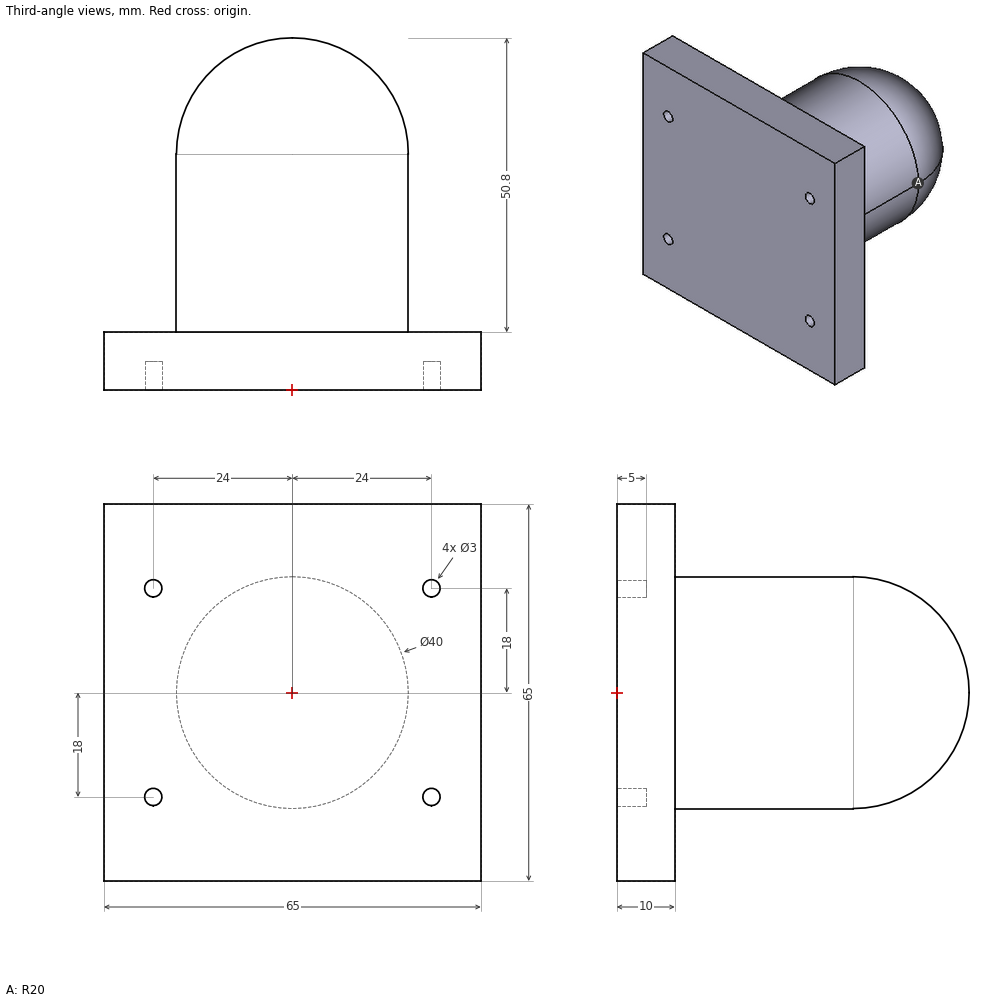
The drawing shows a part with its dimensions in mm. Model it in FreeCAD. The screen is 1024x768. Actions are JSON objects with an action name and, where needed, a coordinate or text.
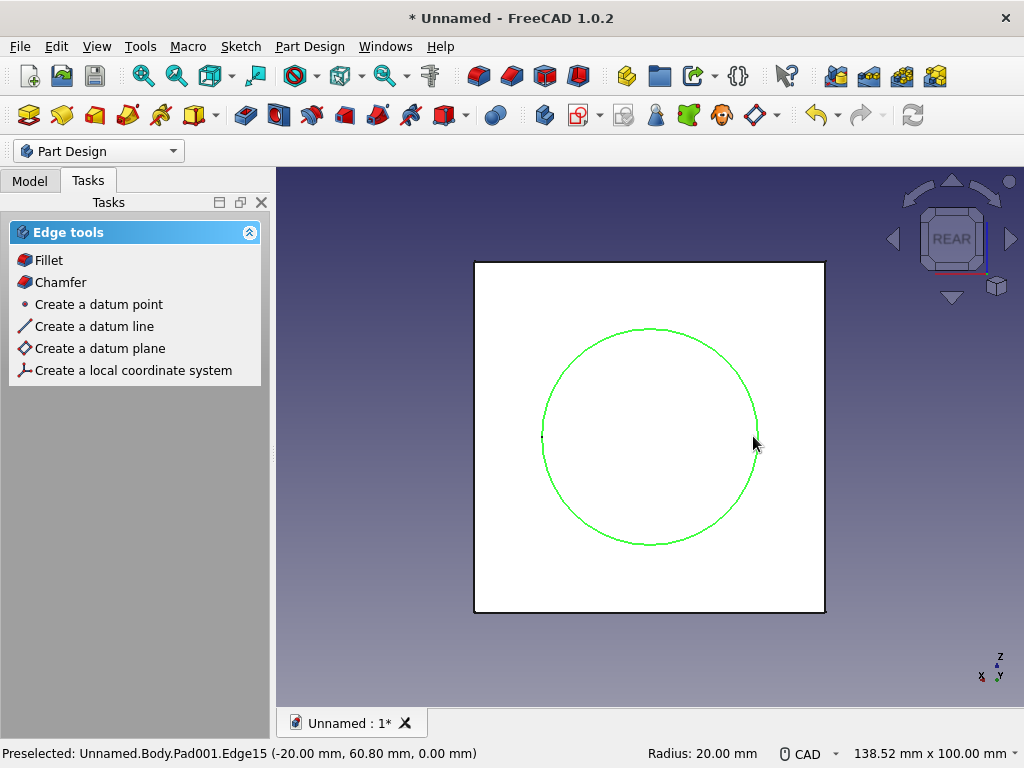
{"action": "left_click", "coordinate": [479, 76]}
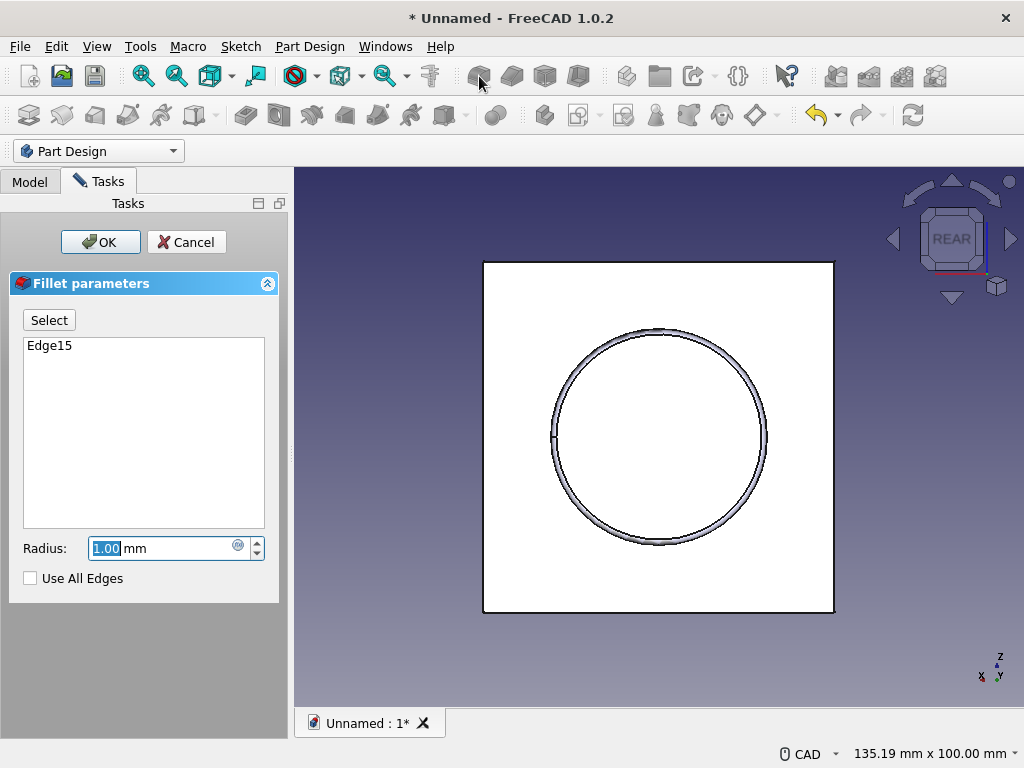
{"action": "type", "text": "20"}
{"action": "key", "text": "Tab"}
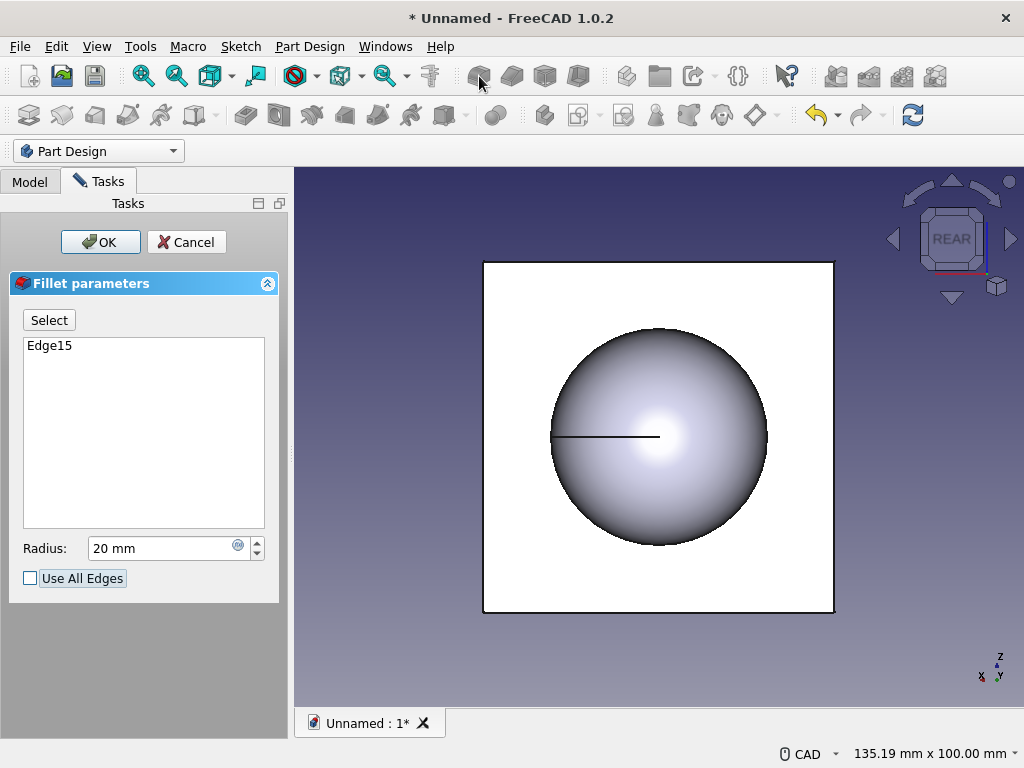
{"action": "left_click", "coordinate": [101, 242]}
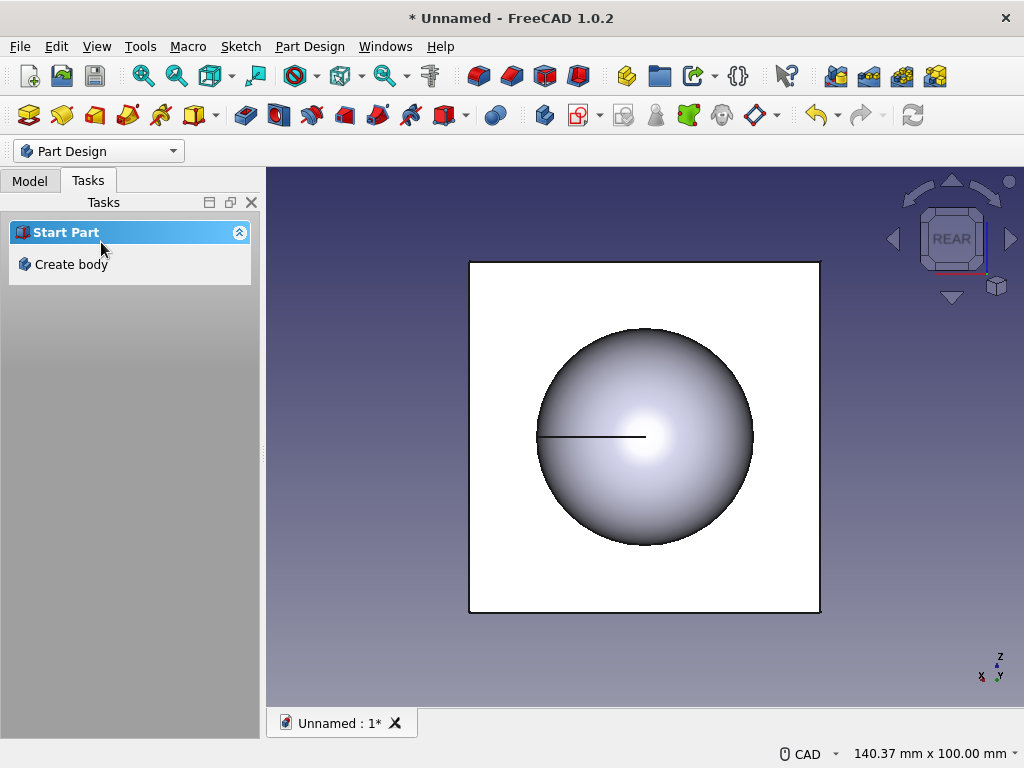
{"action": "left_click", "coordinate": [578, 116]}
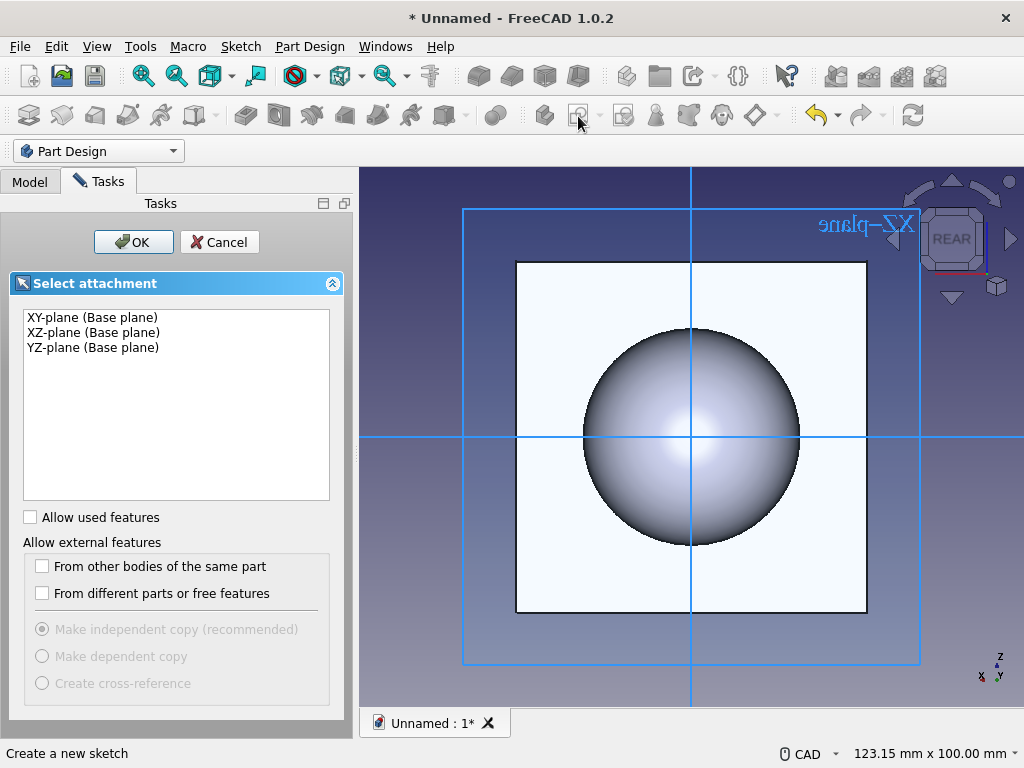
{"action": "left_click", "coordinate": [84, 332]}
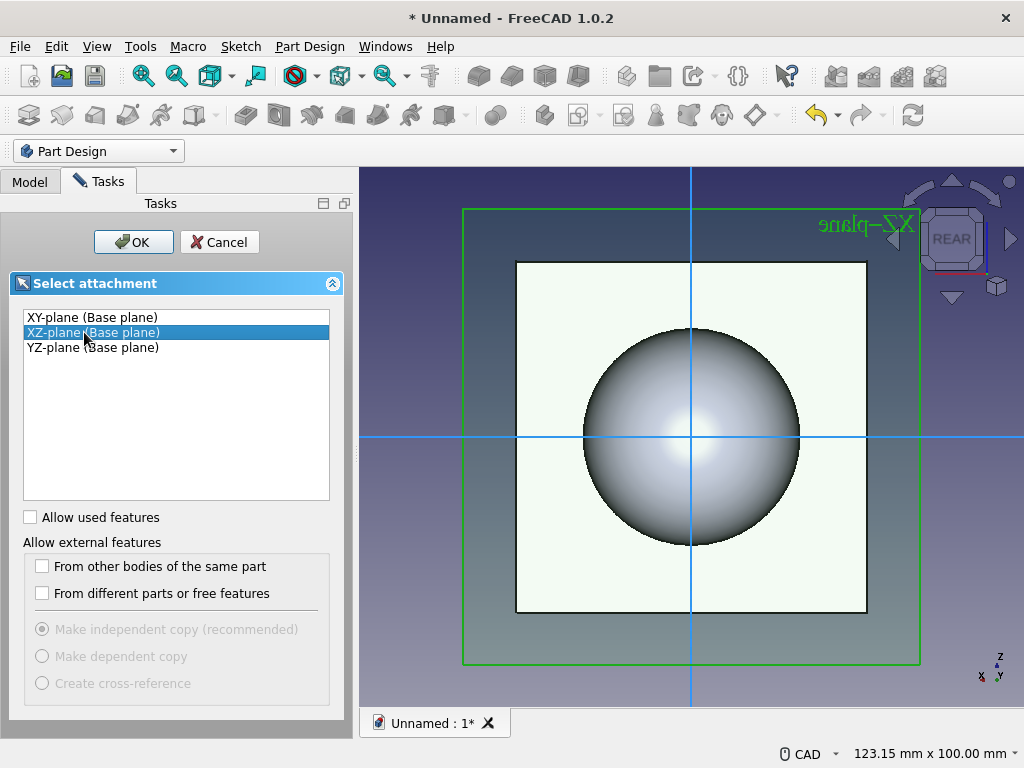
{"action": "left_click", "coordinate": [134, 242]}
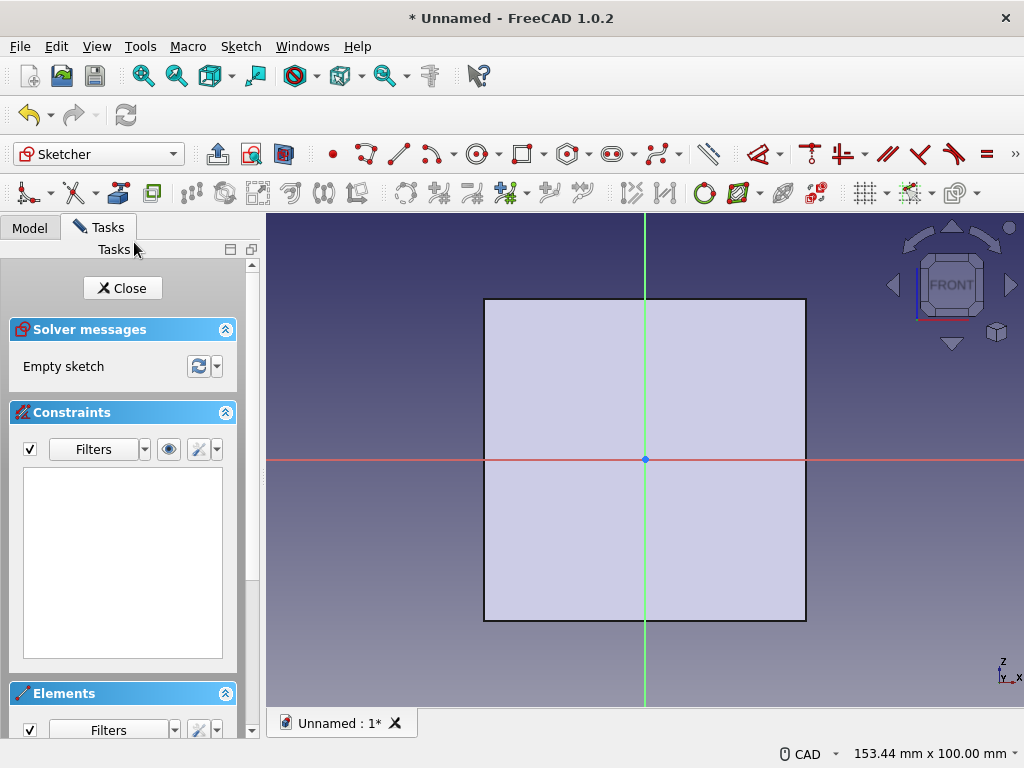
{"action": "scroll", "coordinate": [784, 460], "scroll_direction": "up", "scroll_amount": 2}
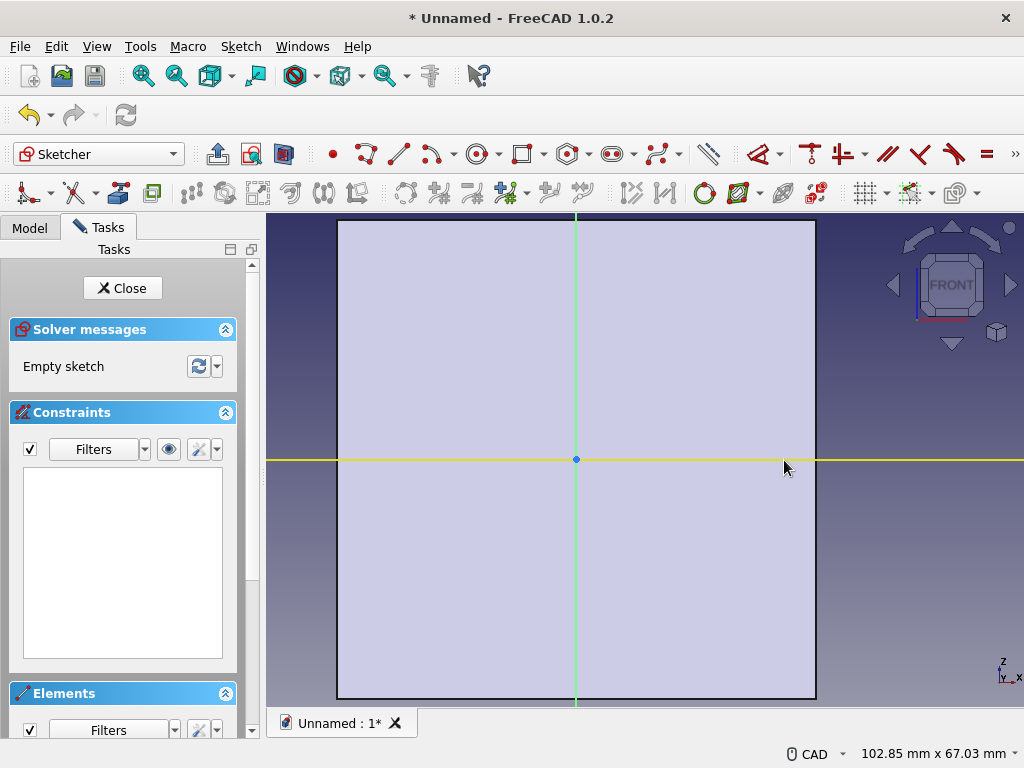
{"action": "left_click", "coordinate": [476, 154]}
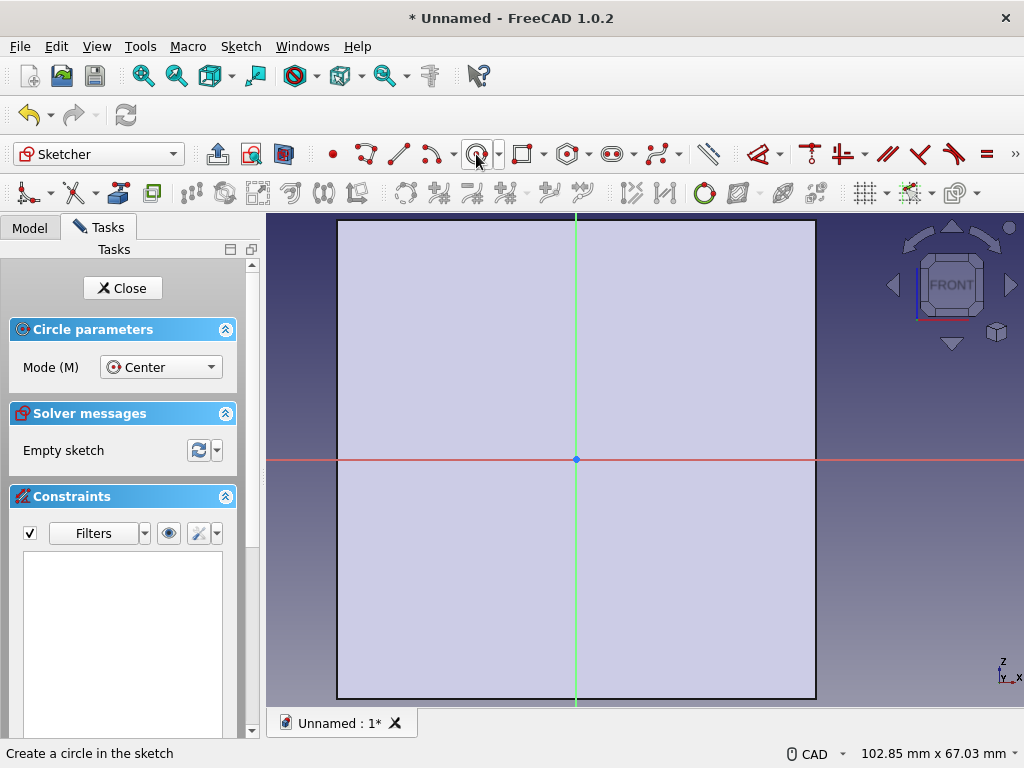
{"action": "scroll", "coordinate": [753, 327], "scroll_direction": "up", "scroll_amount": 4}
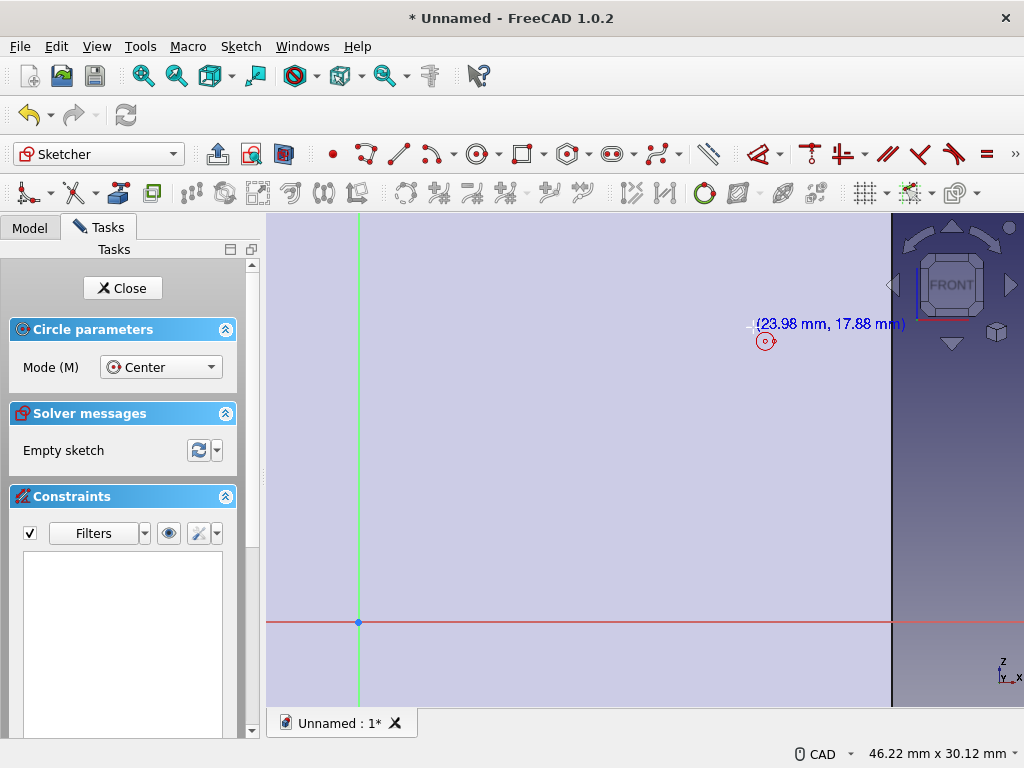
{"action": "left_click", "coordinate": [753, 327]}
{"action": "mouse_move", "coordinate": [770, 310]}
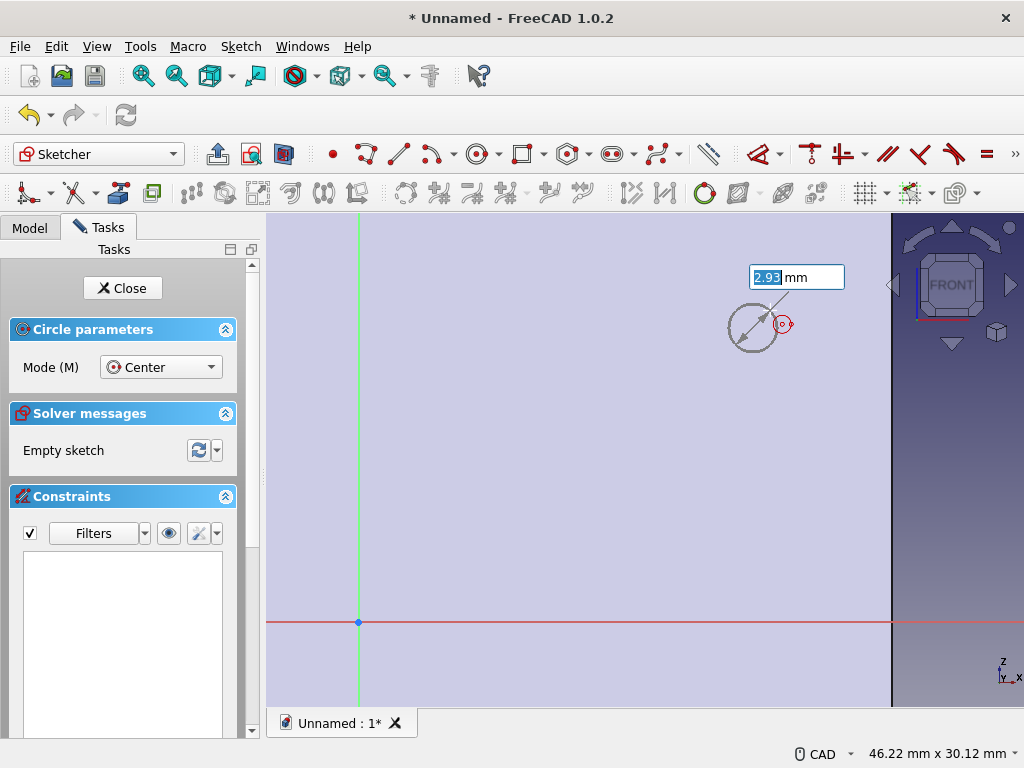
{"action": "type", "text": "3"}
{"action": "key", "text": "Return"}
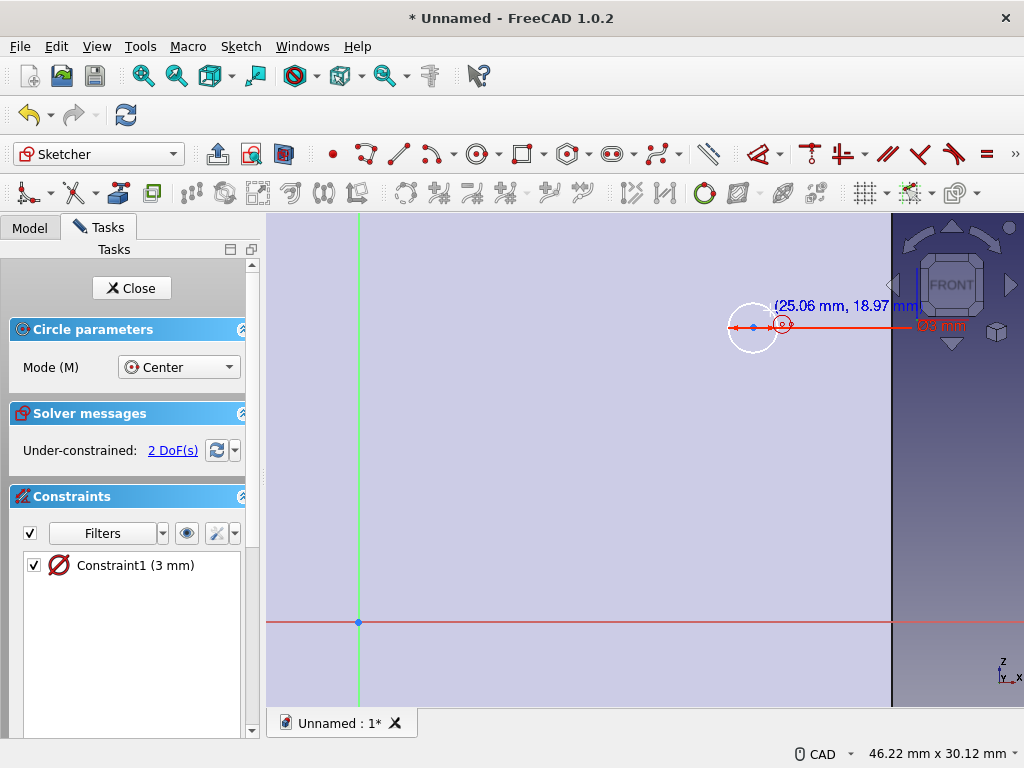
{"action": "scroll", "coordinate": [754, 328], "scroll_direction": "down", "scroll_amount": 4}